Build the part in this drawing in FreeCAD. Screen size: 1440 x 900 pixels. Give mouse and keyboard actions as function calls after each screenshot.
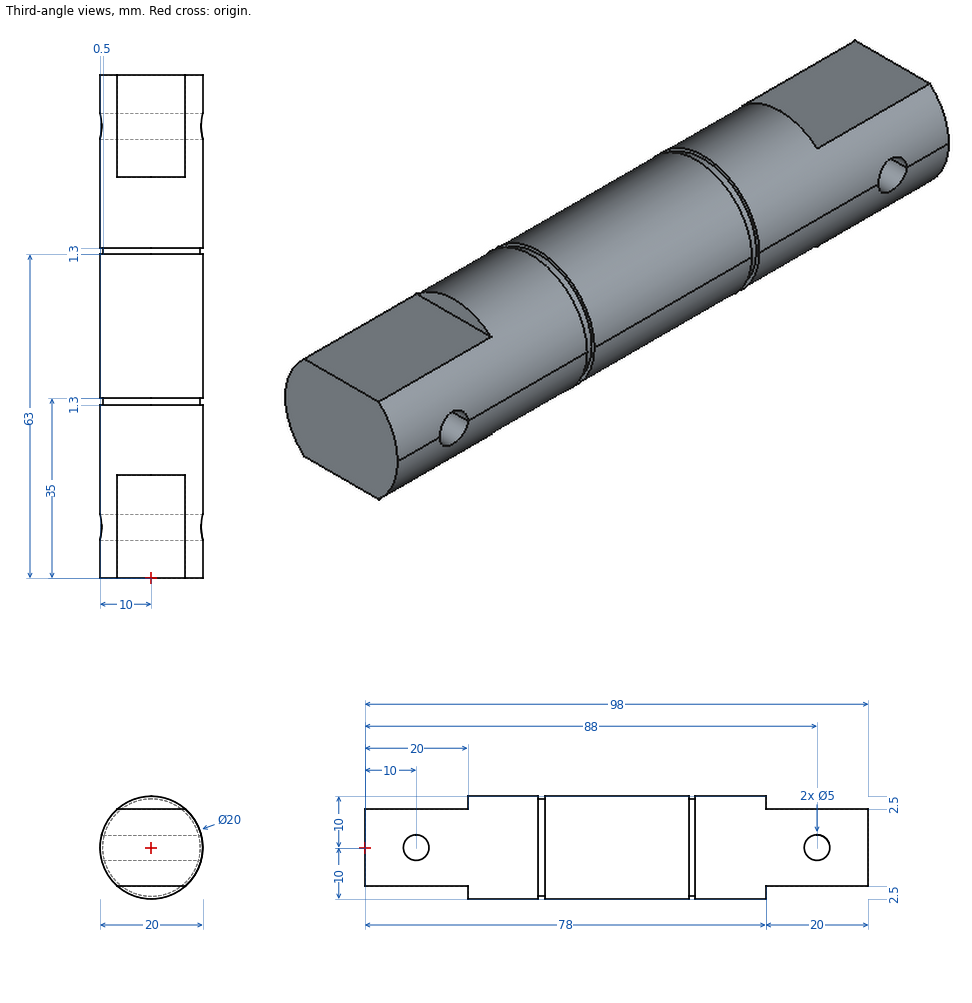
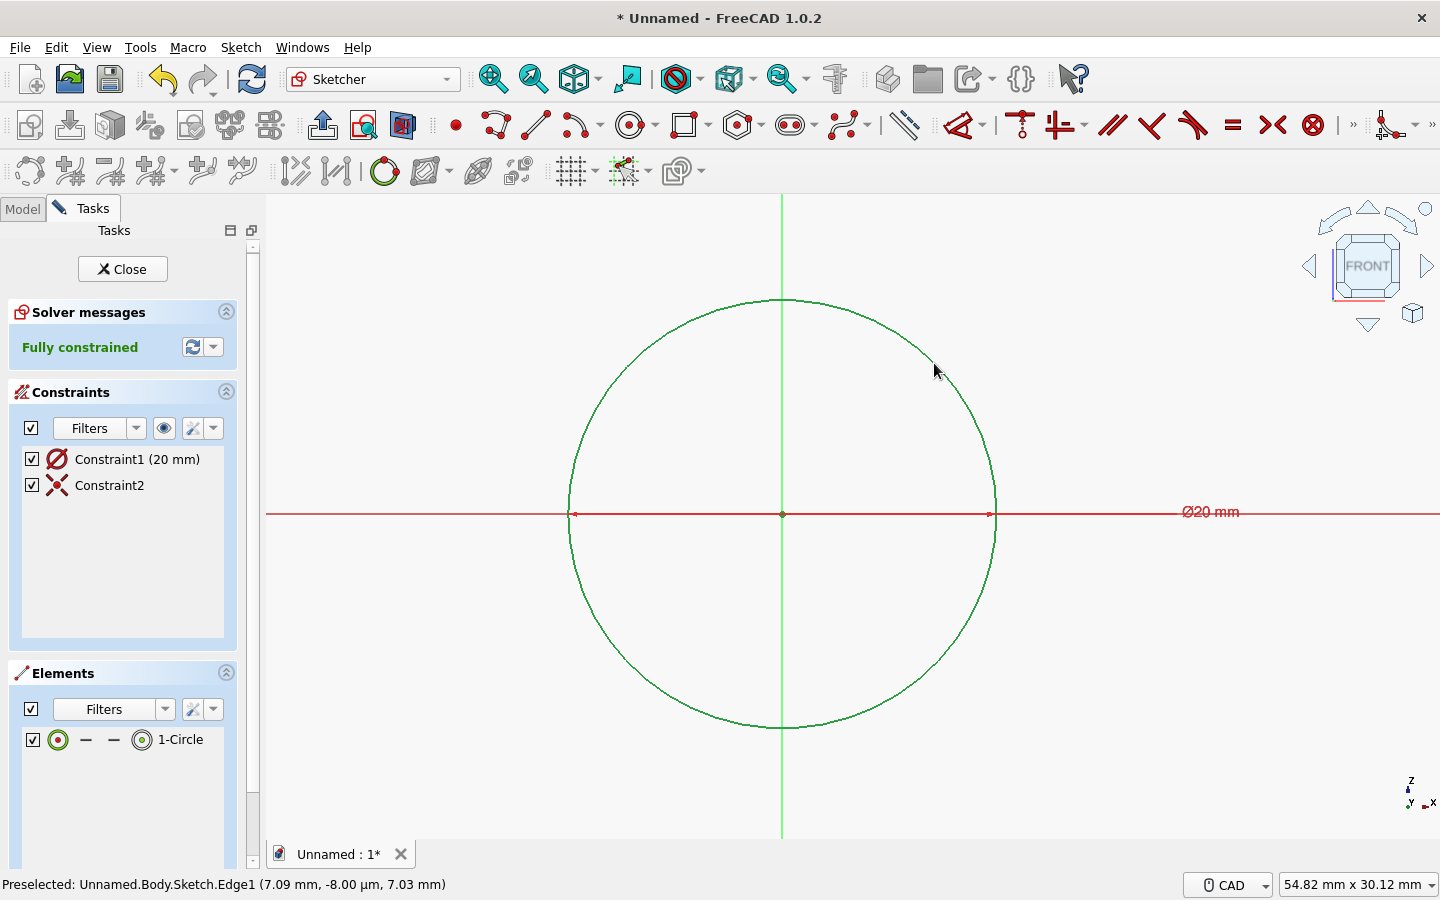
click(123, 269)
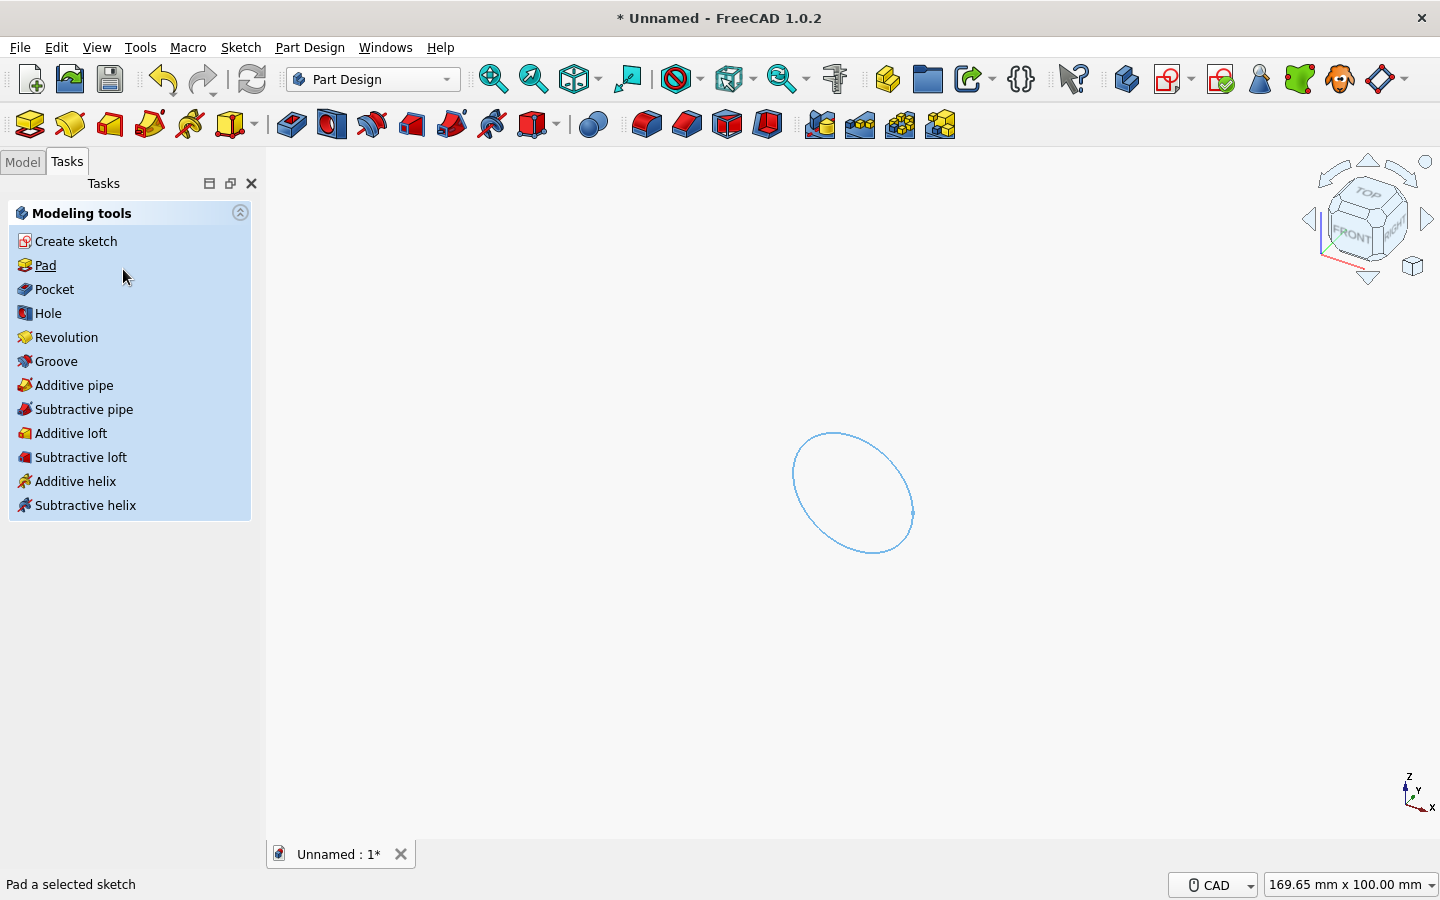
click(30, 124)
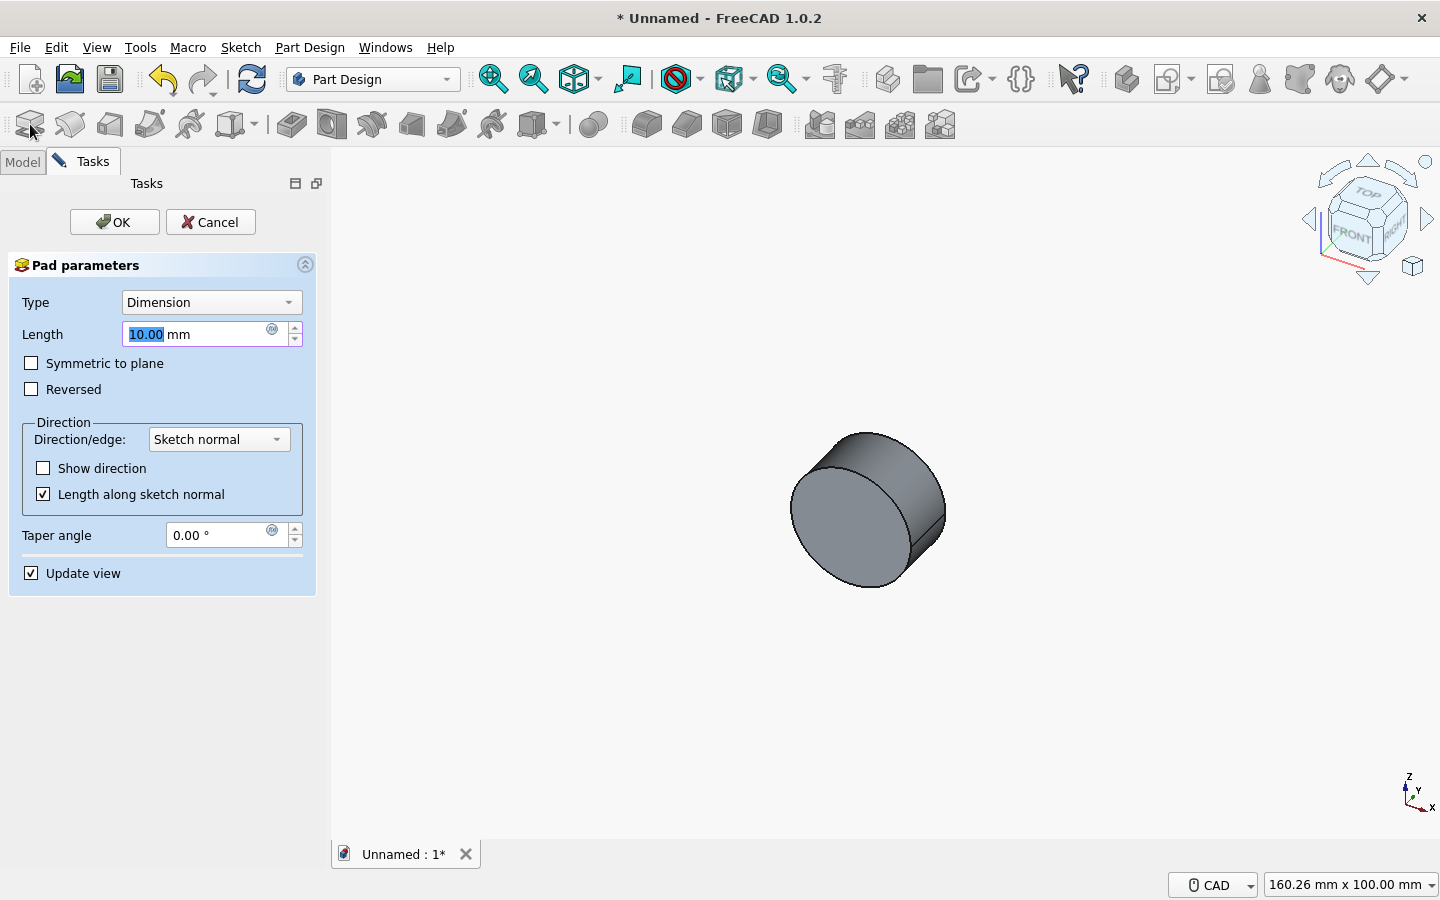
text(98)
key(Tab)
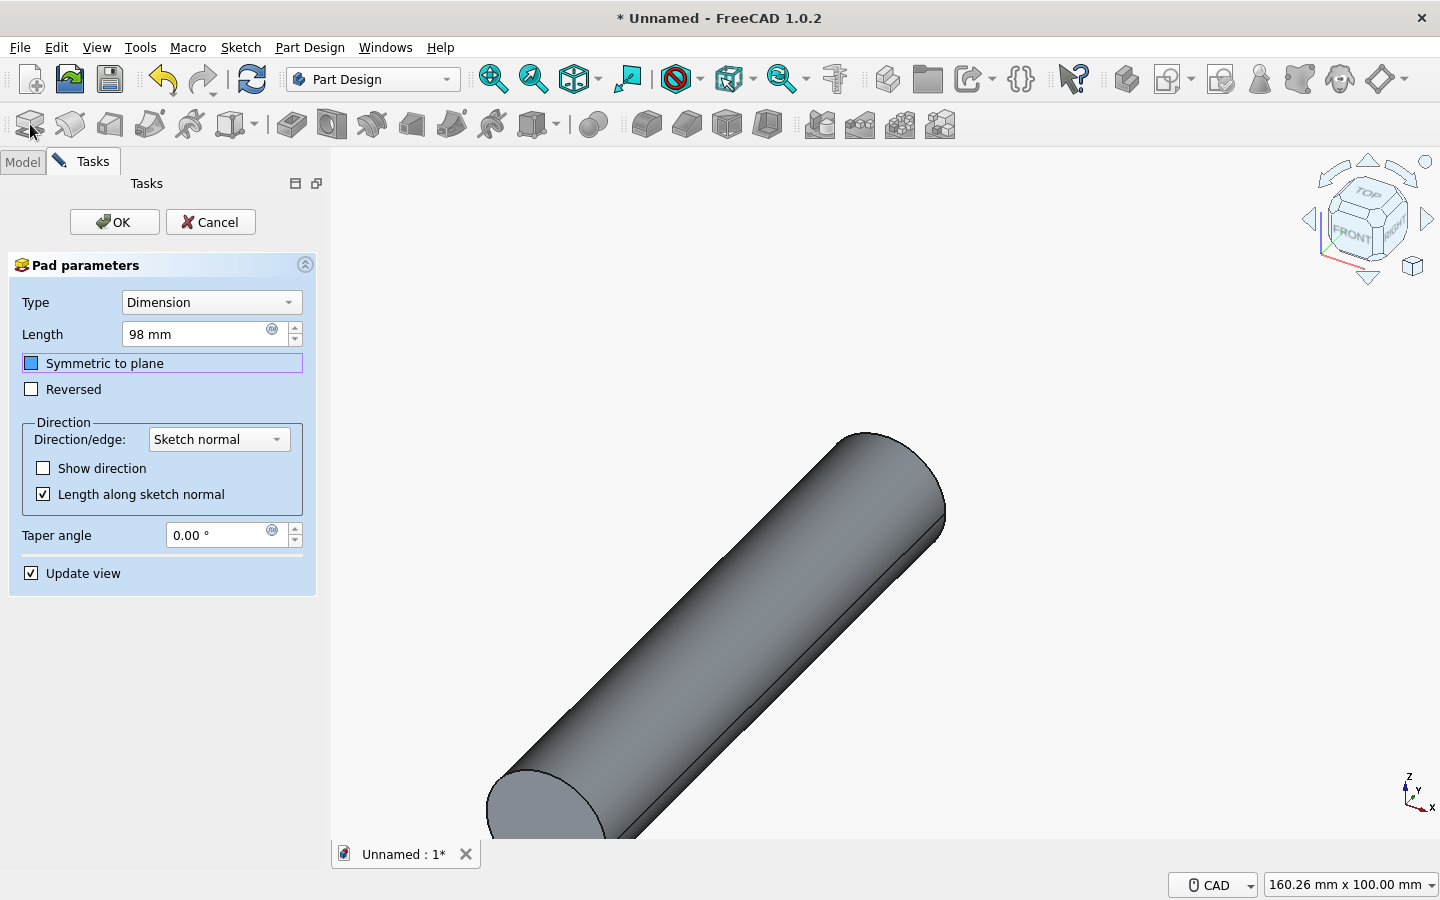
click(30, 389)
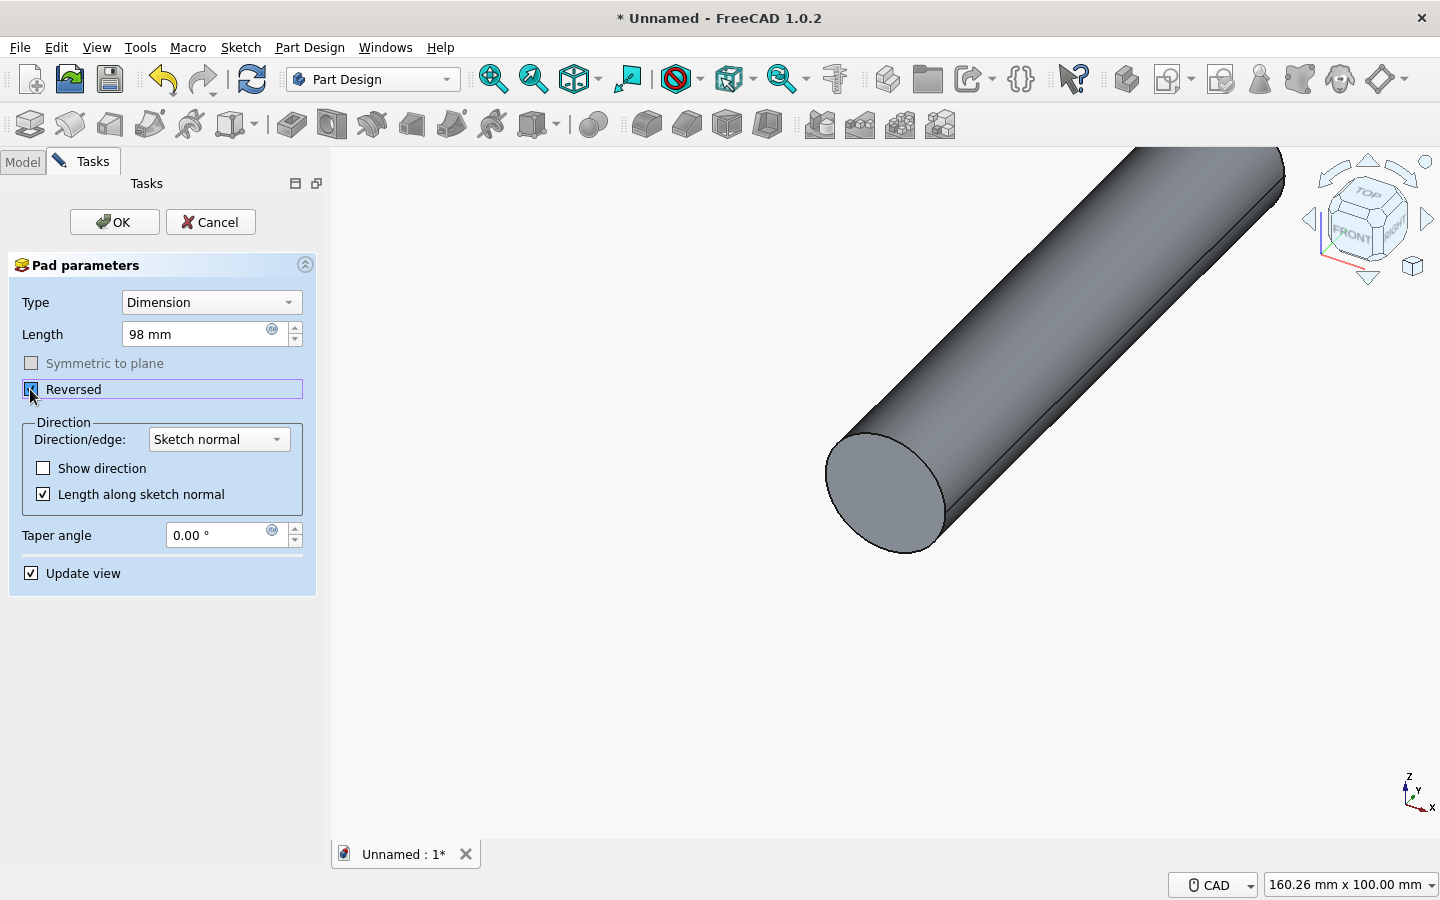
click(115, 222)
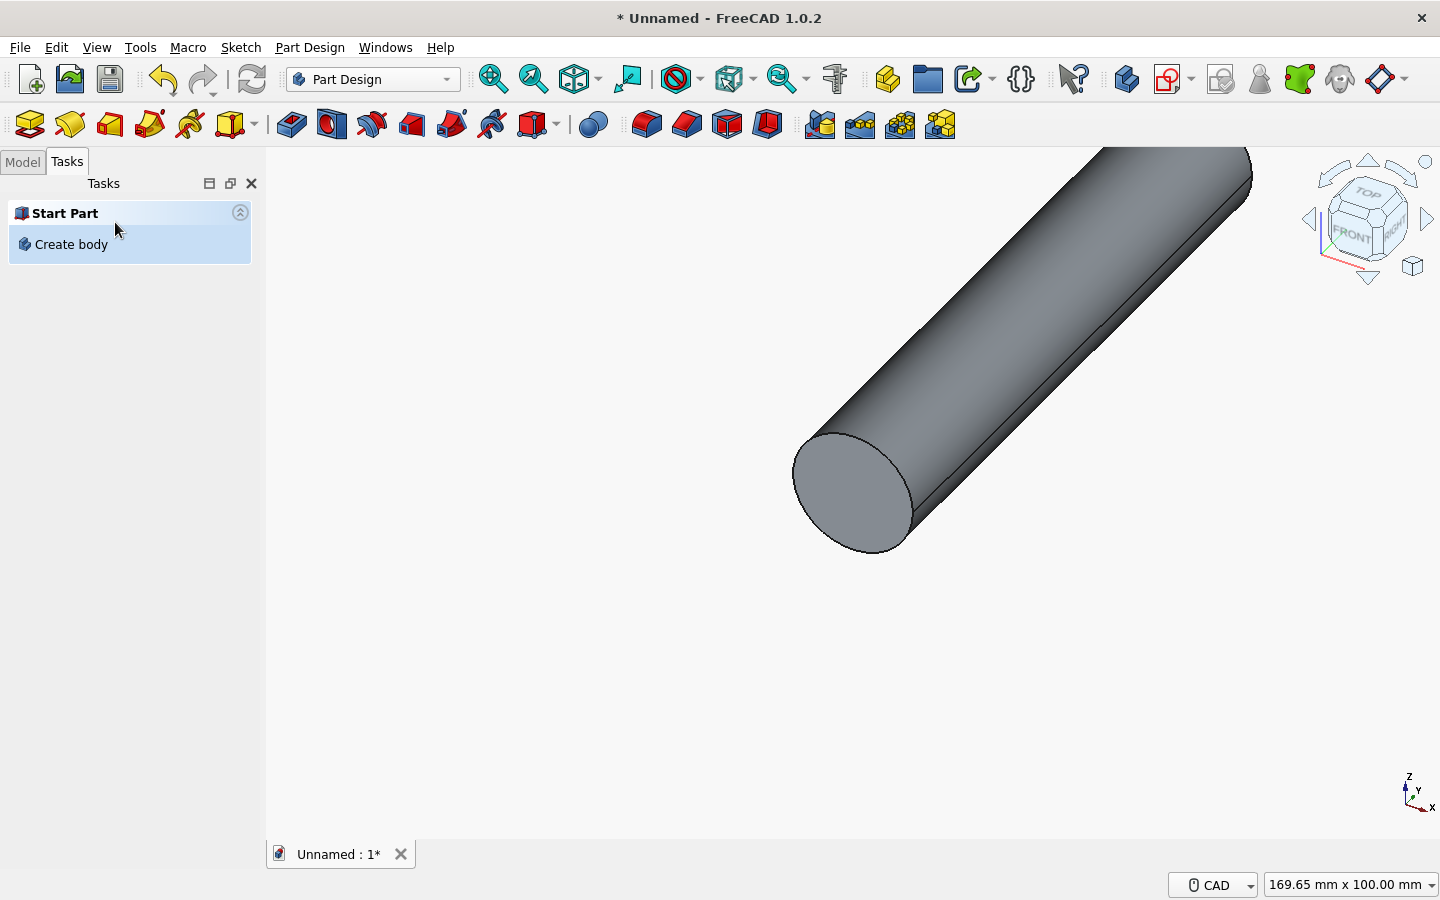
key(v)
key(f)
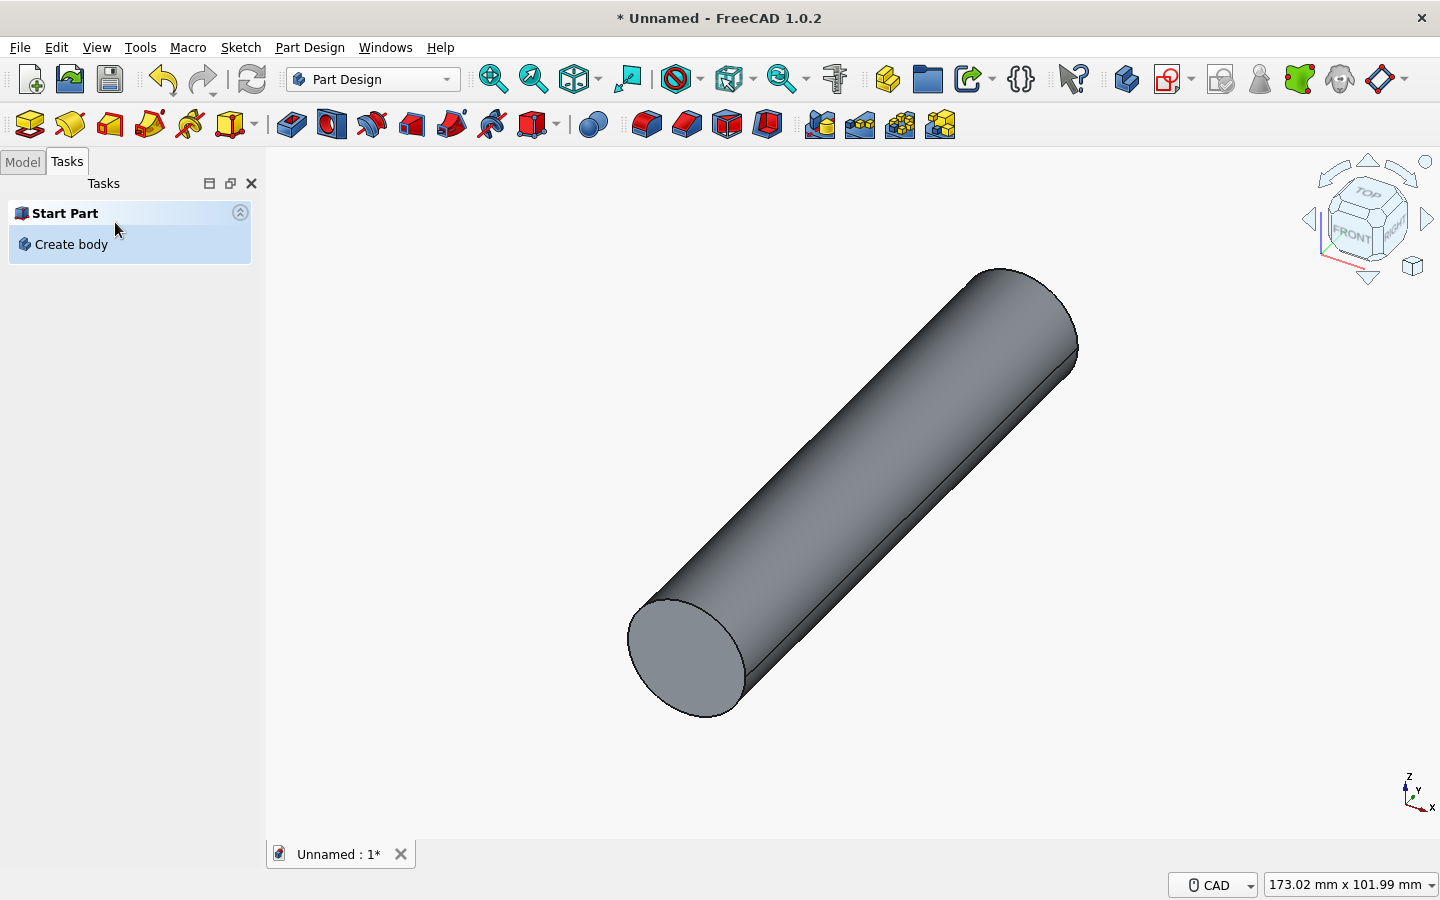
click(1168, 80)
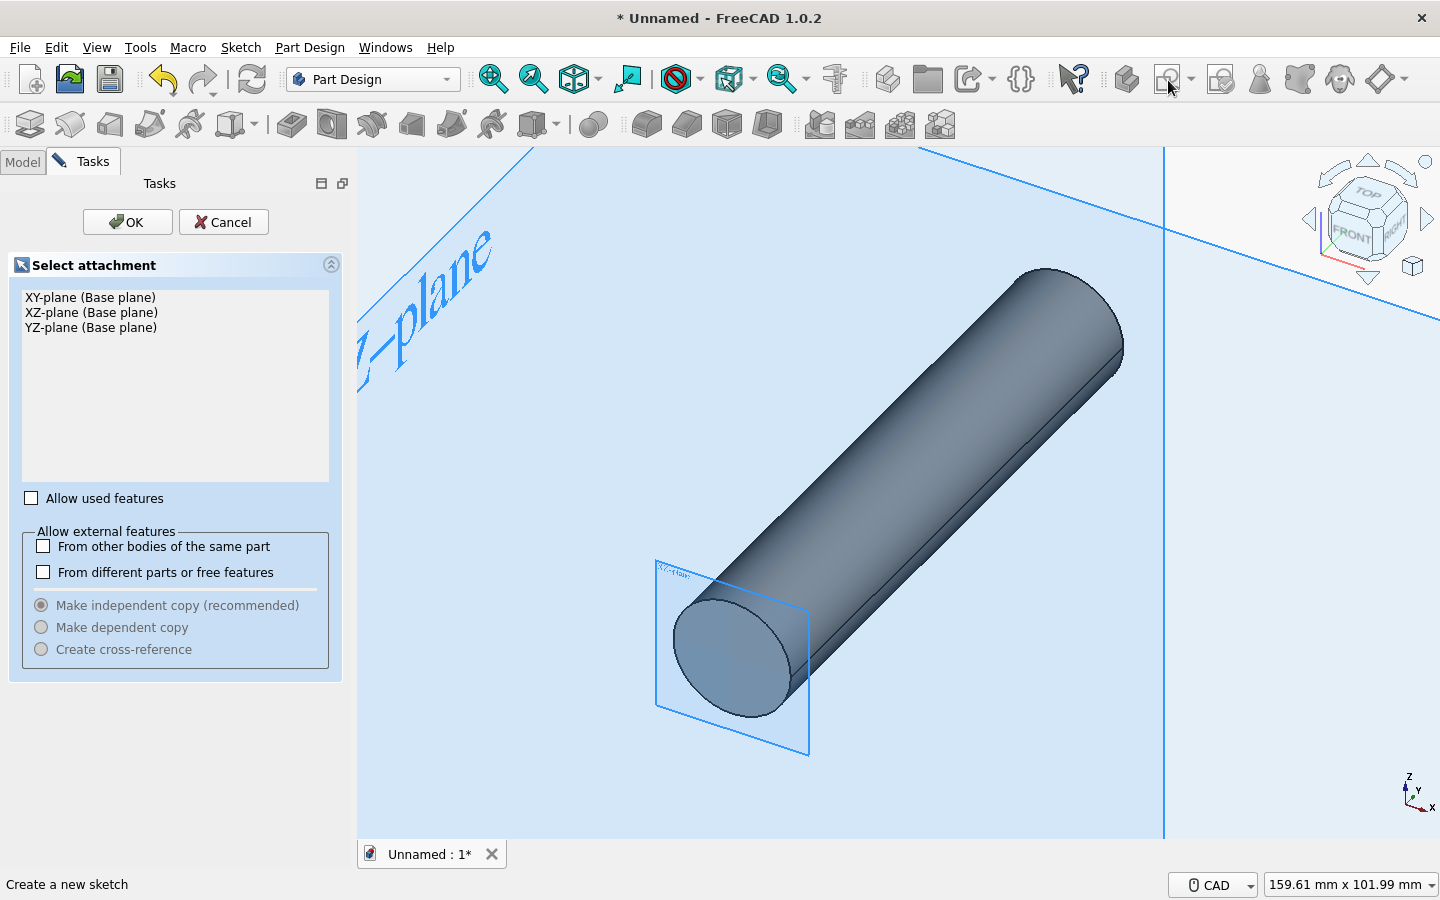
click(82, 328)